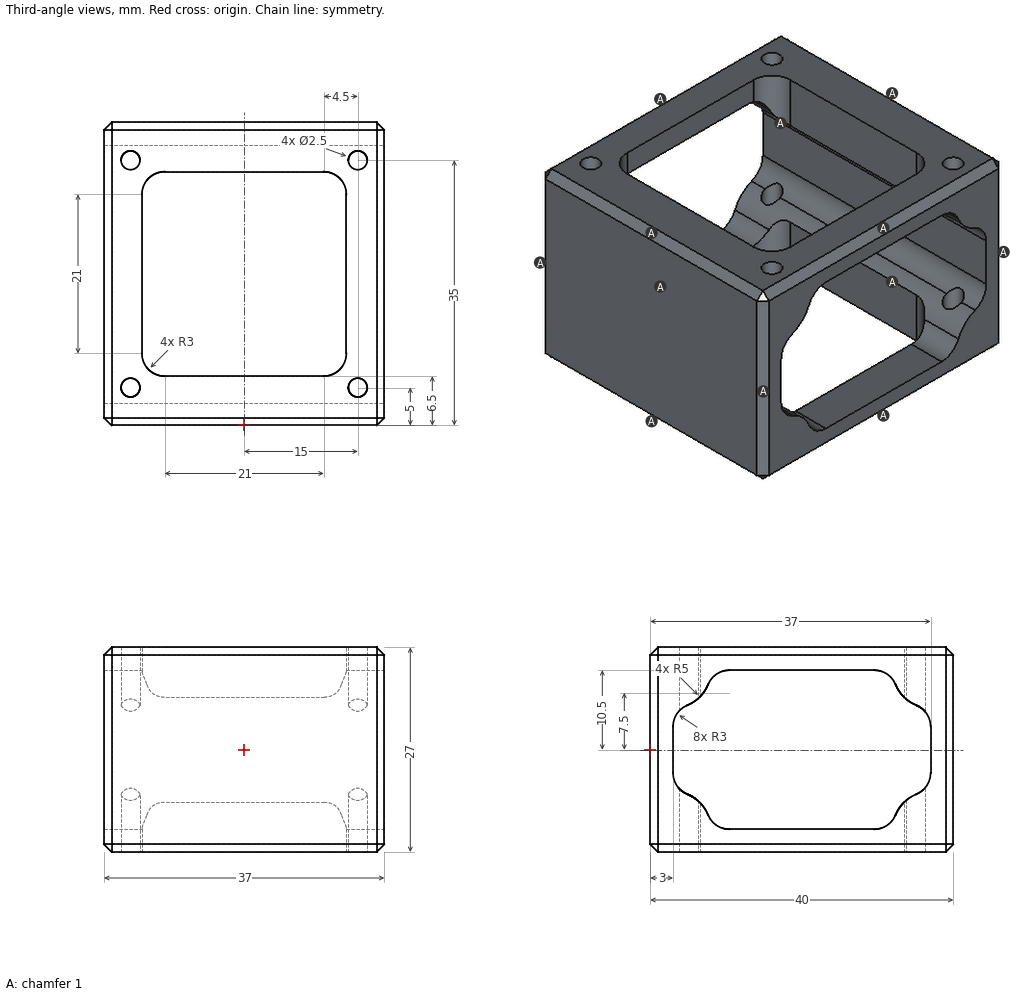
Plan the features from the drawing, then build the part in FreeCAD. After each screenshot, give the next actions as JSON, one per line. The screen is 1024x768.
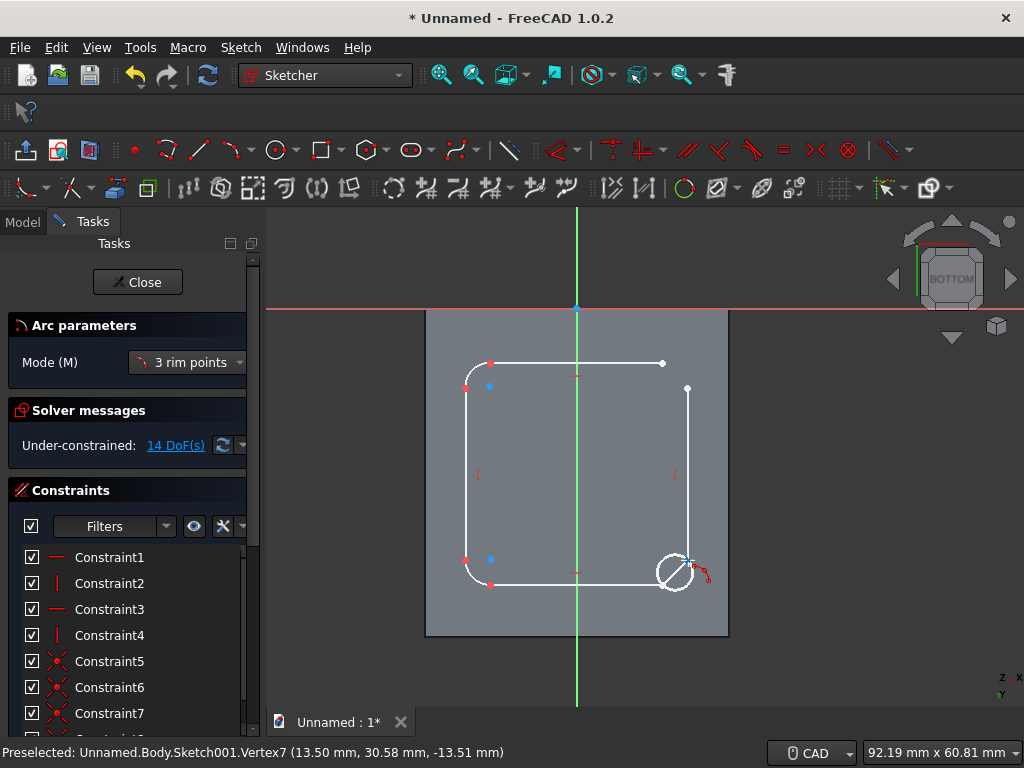
{"action": "scroll", "coordinate": [680, 577], "scroll_direction": "up", "scroll_amount": 4}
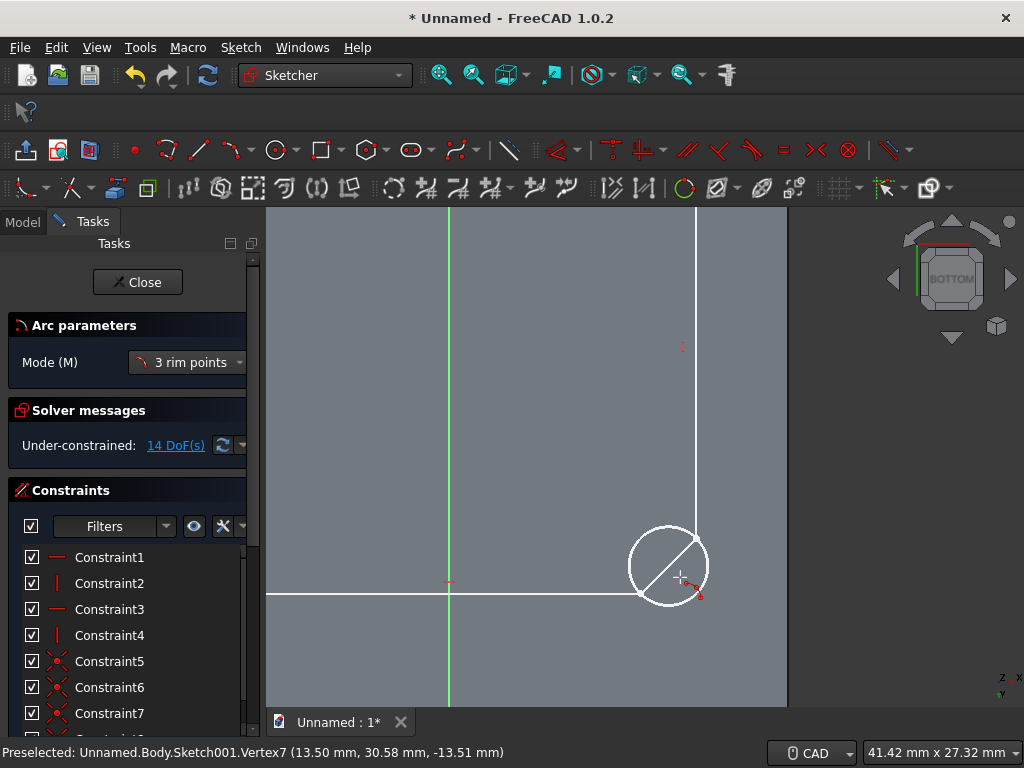
{"action": "left_click", "coordinate": [680, 576]}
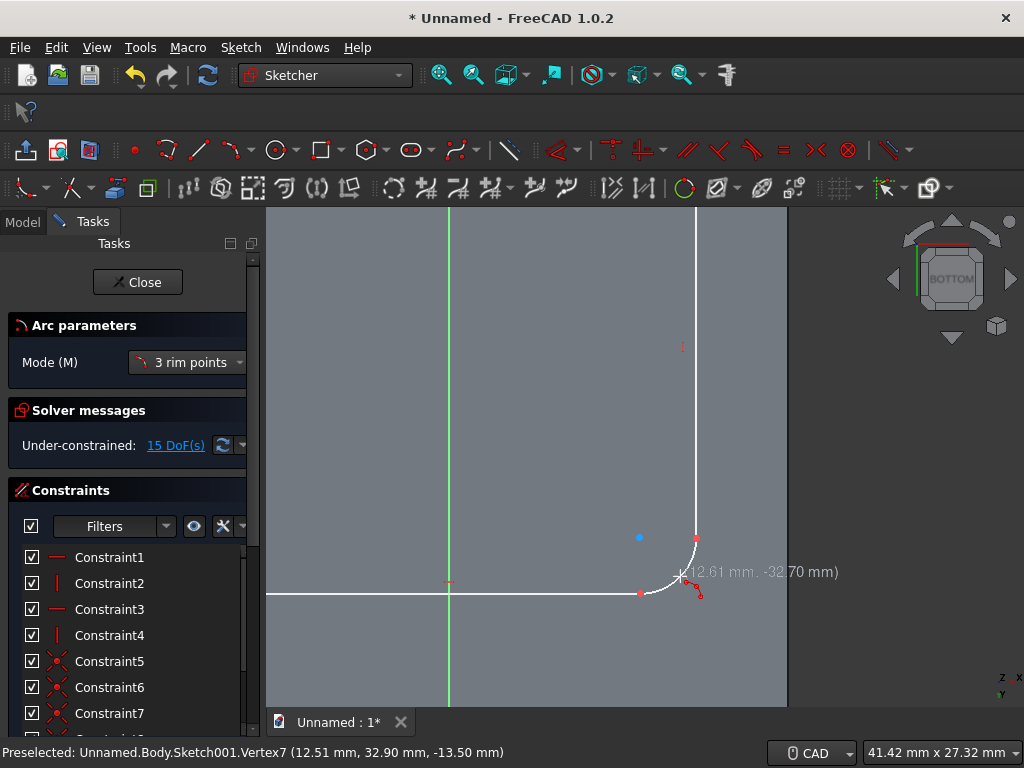
{"action": "scroll", "coordinate": [680, 577], "scroll_direction": "down", "scroll_amount": 4}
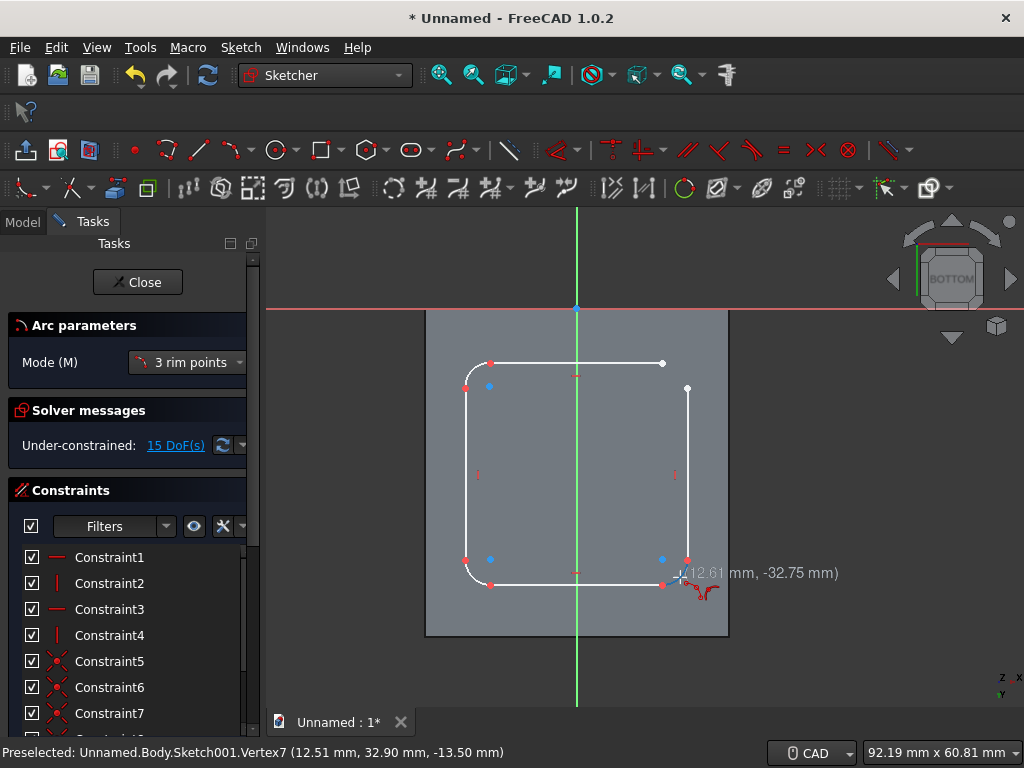
{"action": "left_click", "coordinate": [688, 388]}
{"action": "left_click", "coordinate": [663, 363]}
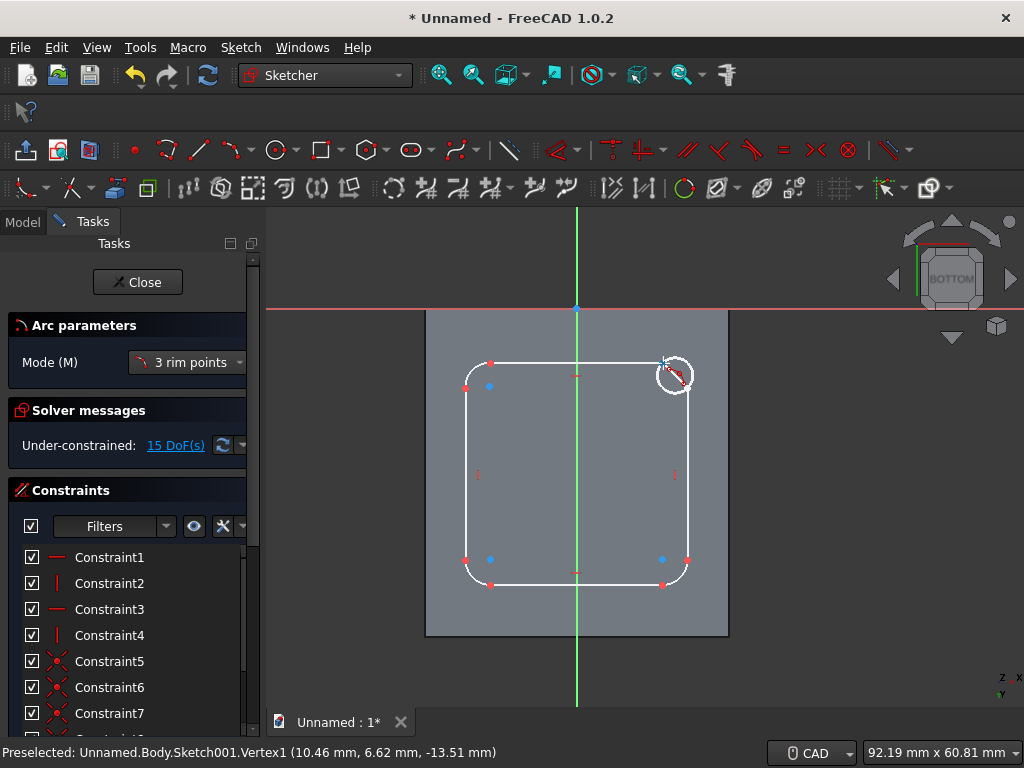
{"action": "scroll", "coordinate": [680, 369], "scroll_direction": "up", "scroll_amount": 4}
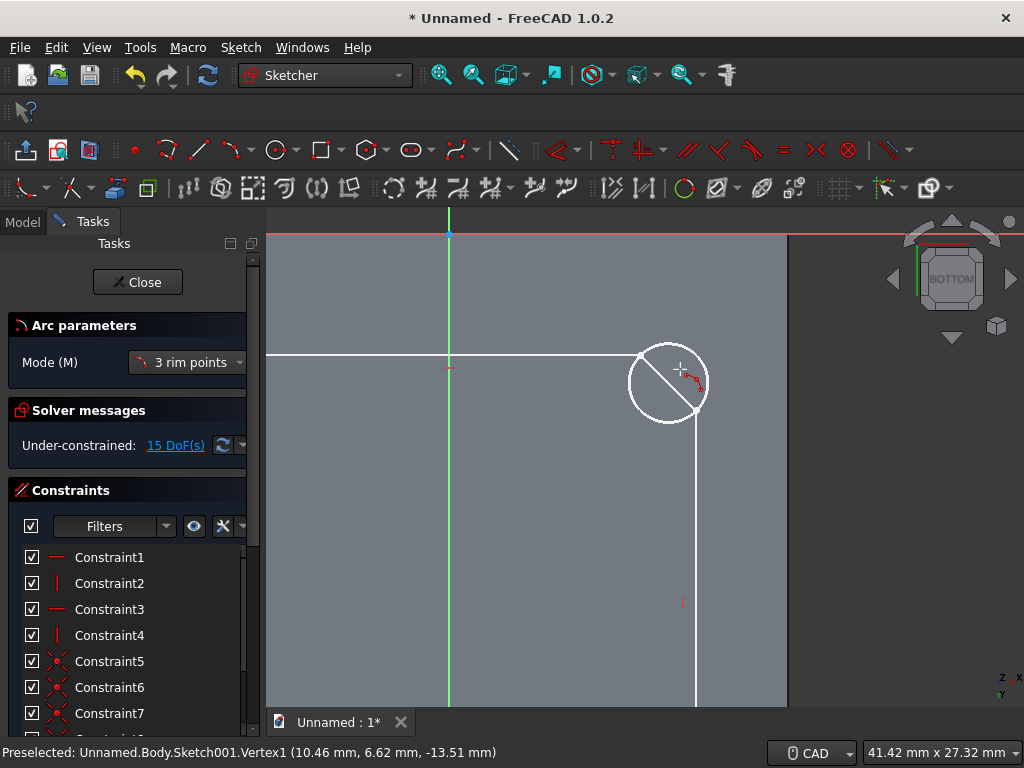
{"action": "left_click", "coordinate": [680, 369]}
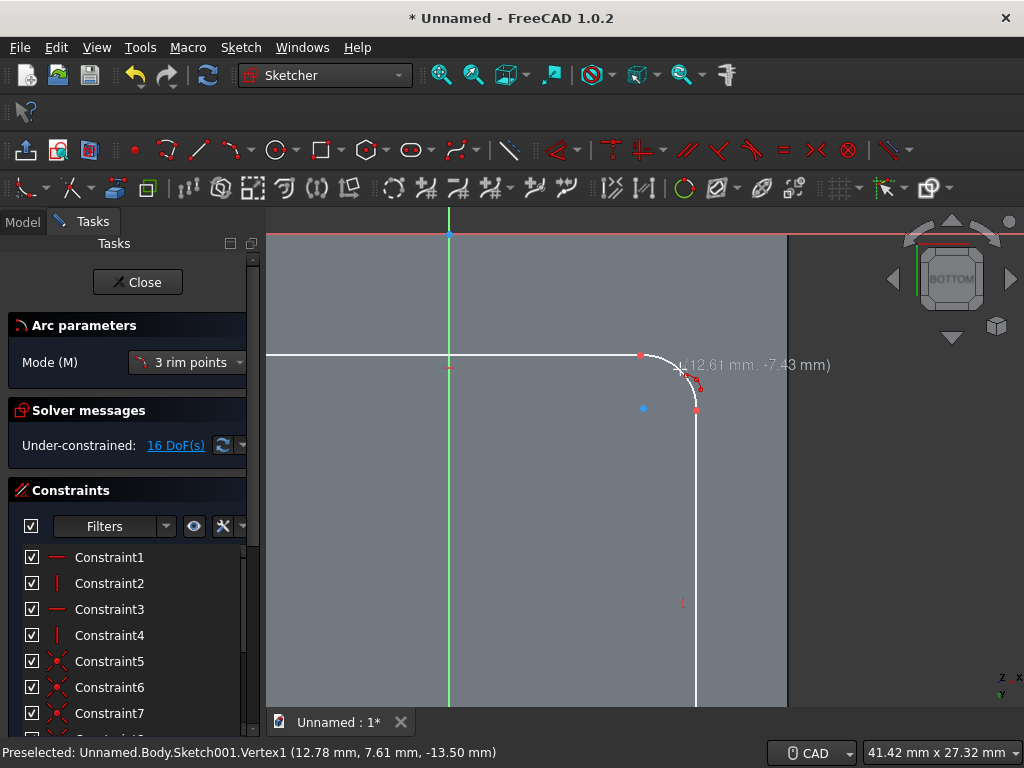
{"action": "key", "text": "g c"}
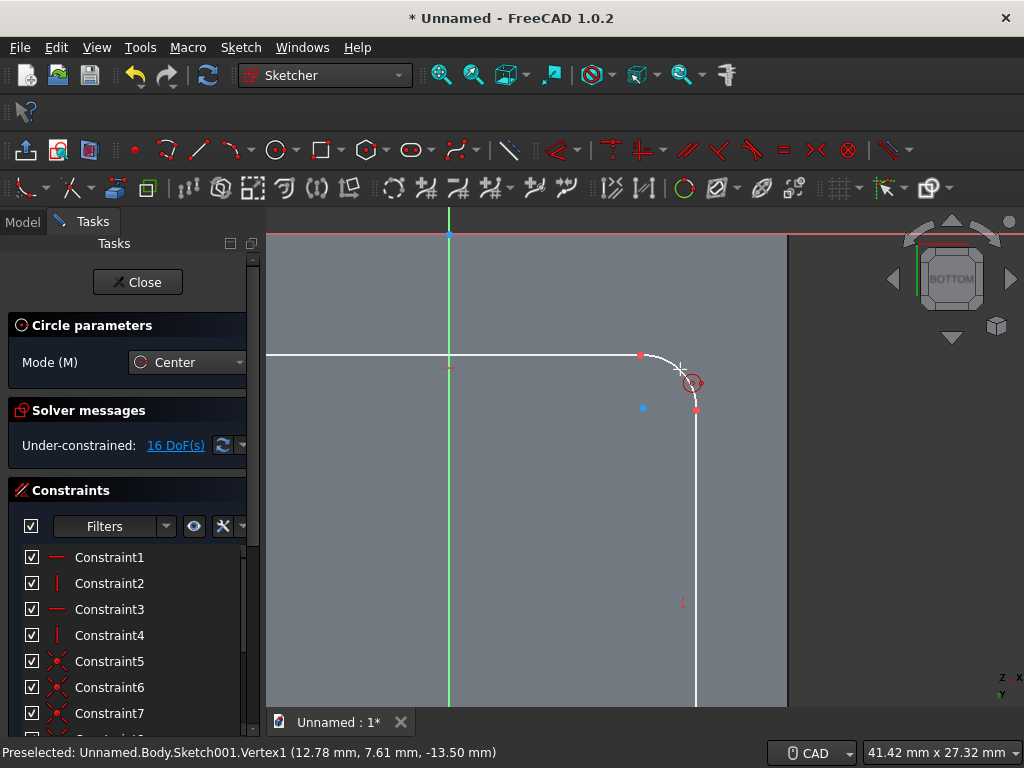
{"action": "scroll", "coordinate": [680, 368], "scroll_direction": "down", "scroll_amount": 4}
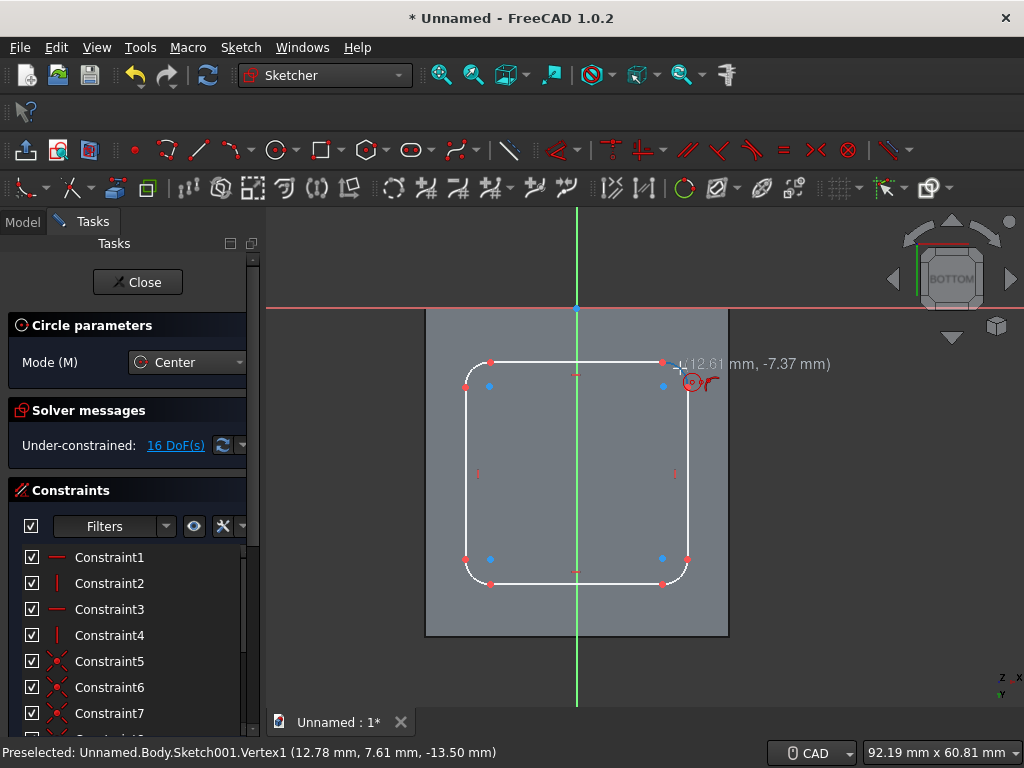
{"action": "scroll", "coordinate": [700, 596], "scroll_direction": "up", "scroll_amount": 4}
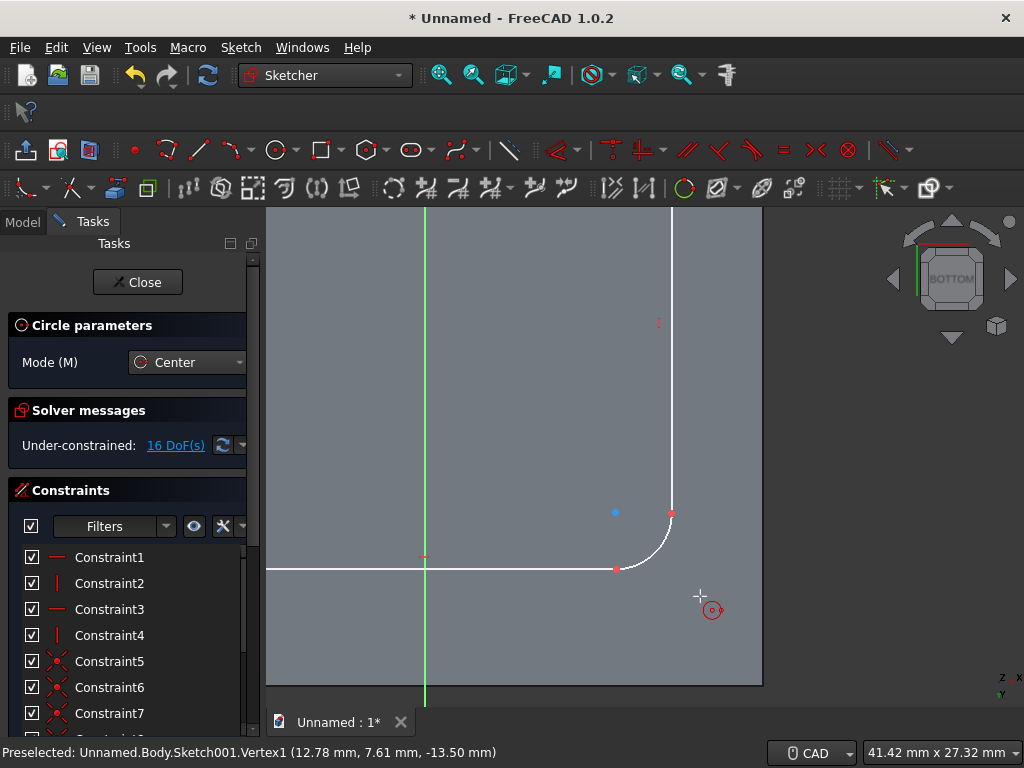
{"action": "left_click", "coordinate": [699, 595]}
{"action": "left_click", "coordinate": [715, 578]}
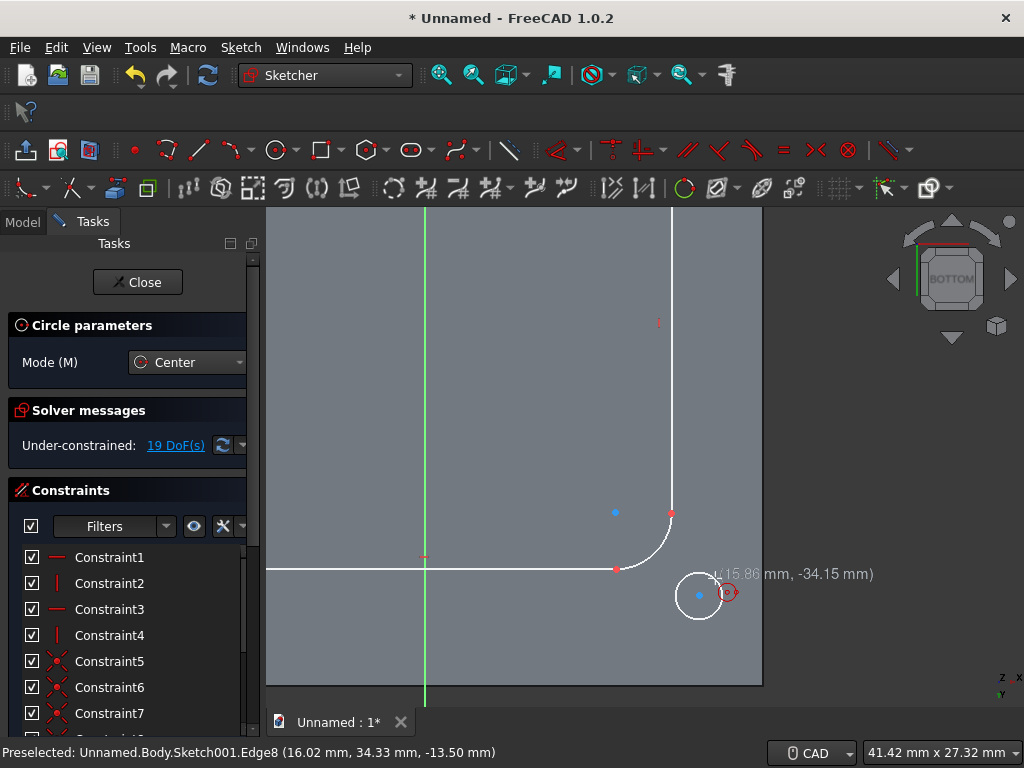
{"action": "scroll", "coordinate": [700, 597], "scroll_direction": "down", "scroll_amount": 4}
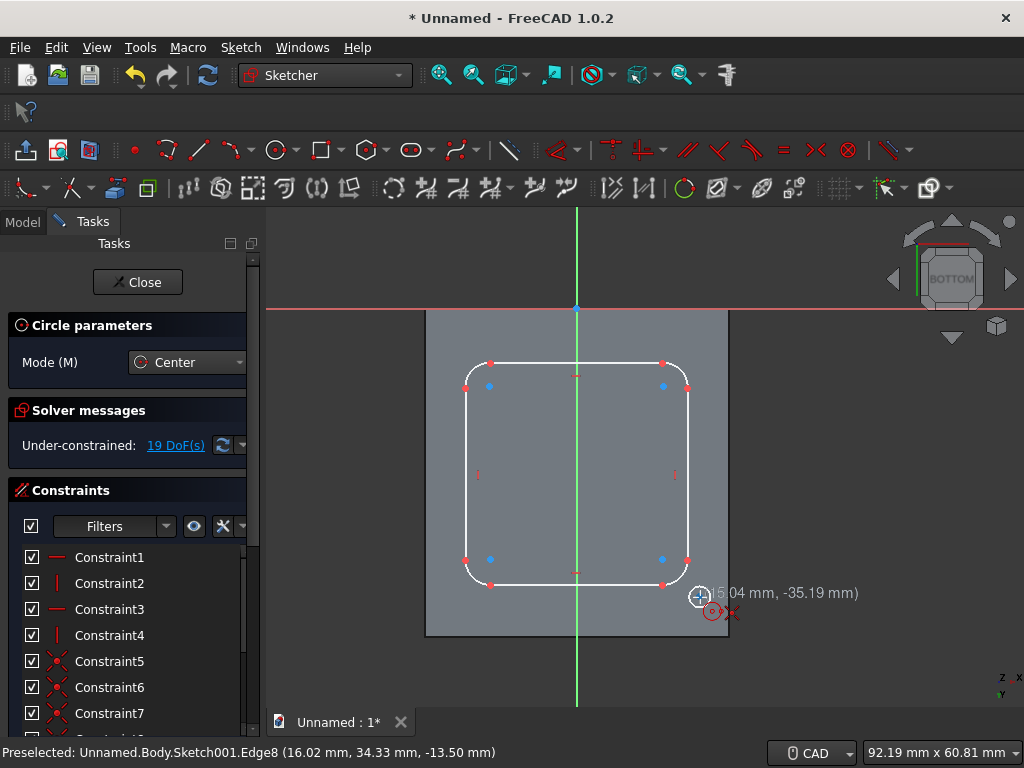
{"action": "scroll", "coordinate": [453, 596], "scroll_direction": "up", "scroll_amount": 4}